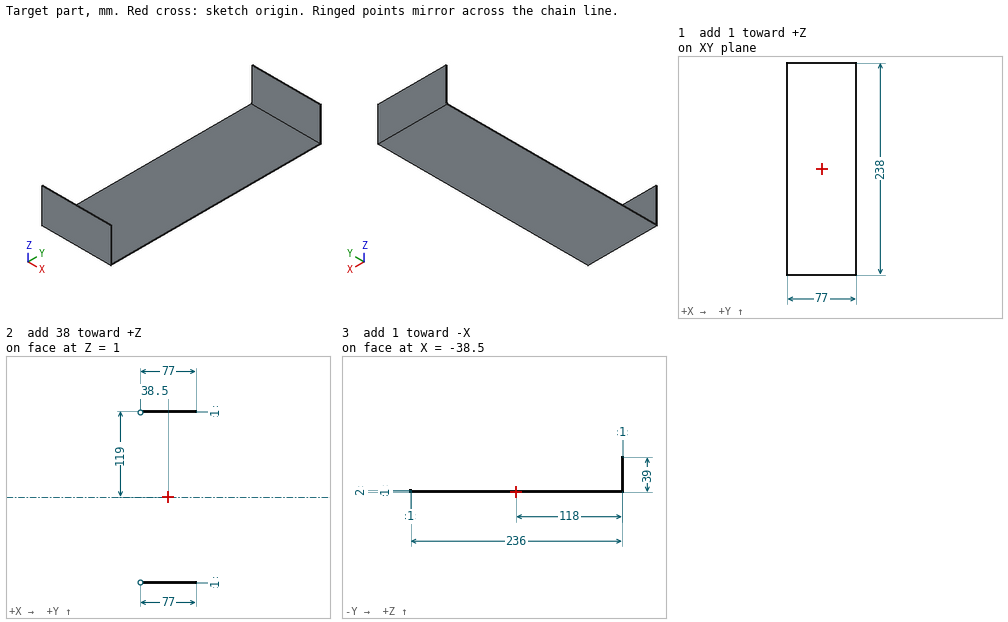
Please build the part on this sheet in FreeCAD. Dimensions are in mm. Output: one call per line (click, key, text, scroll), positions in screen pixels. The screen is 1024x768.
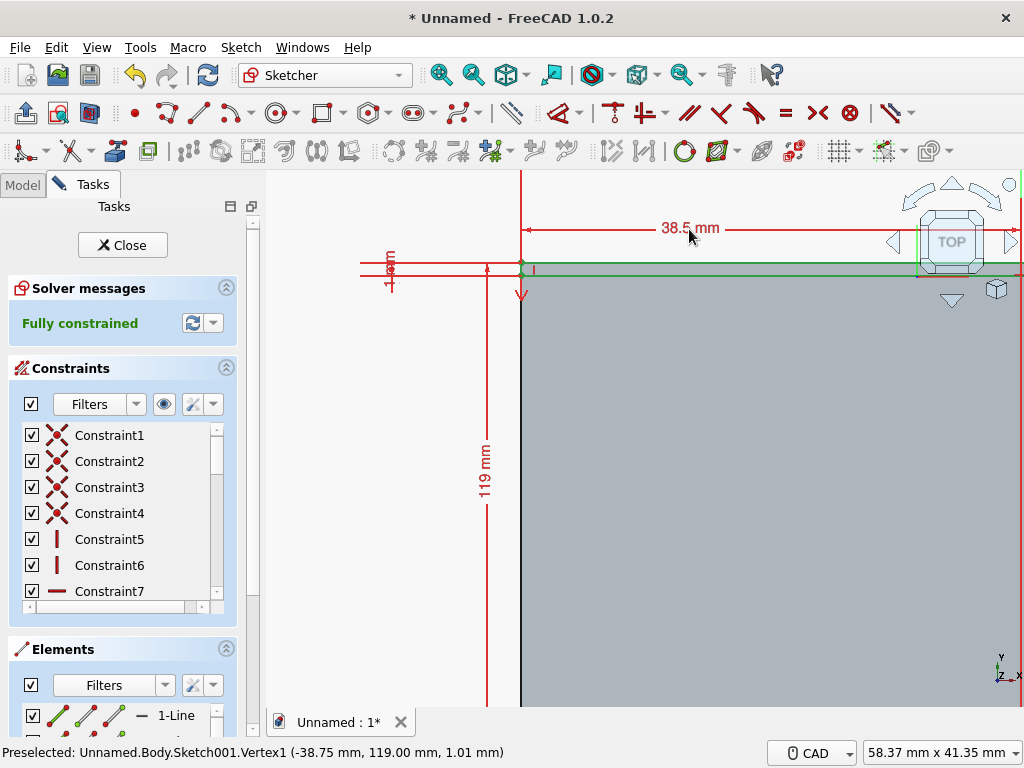
click(123, 245)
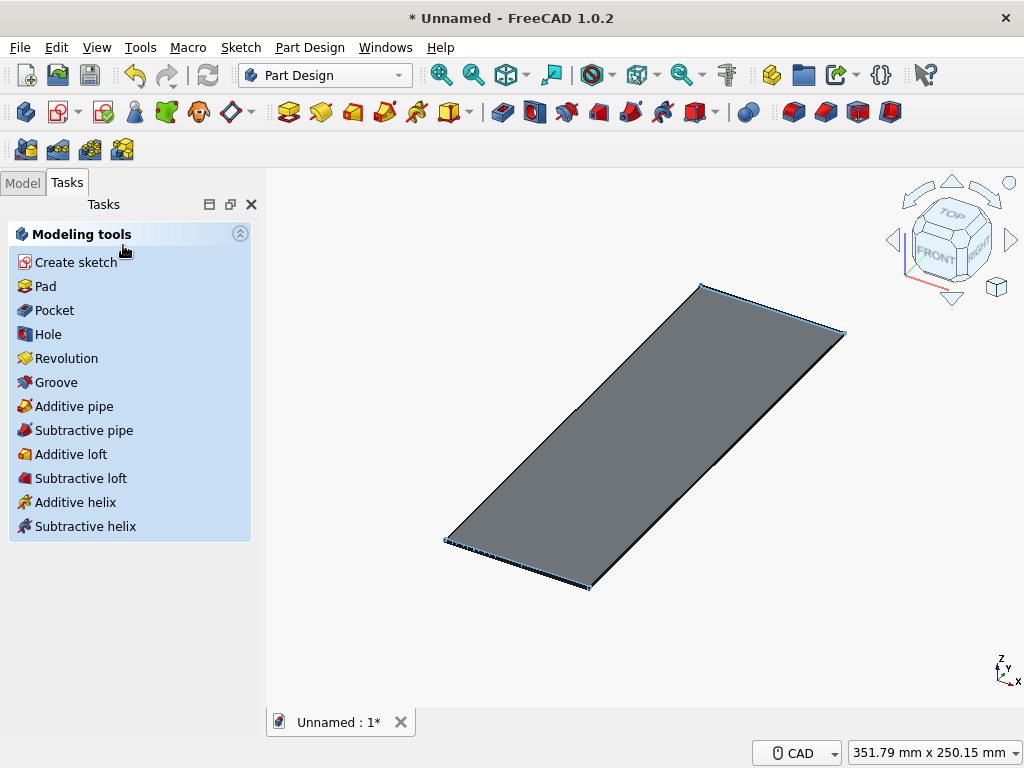
click(290, 112)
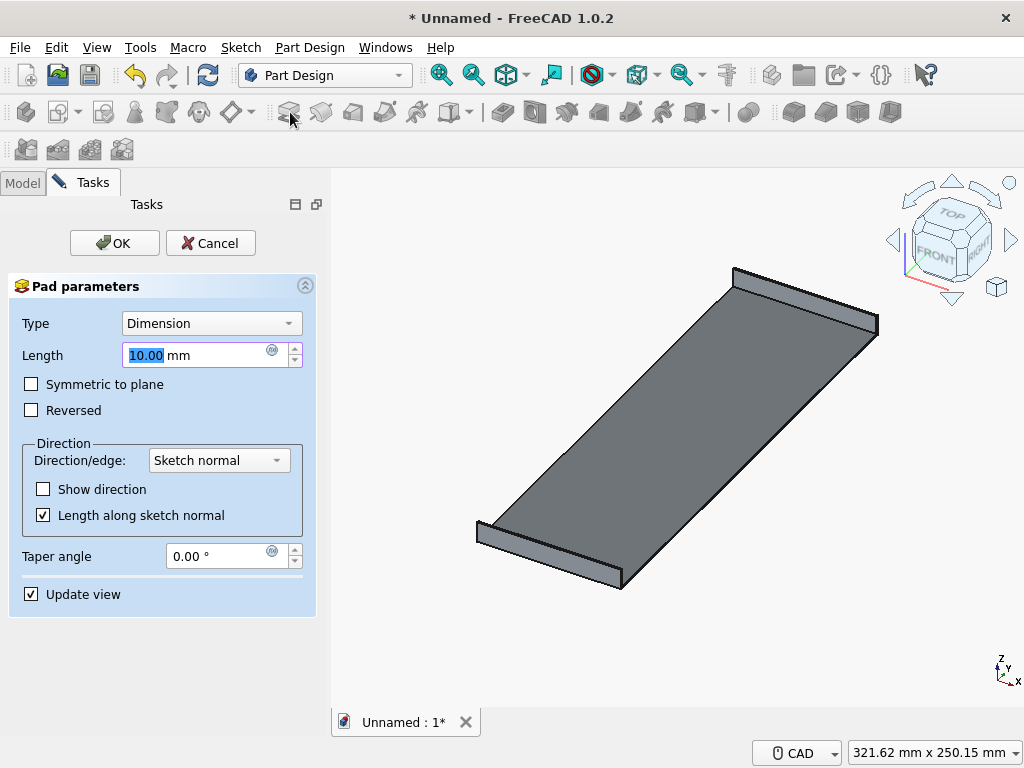
text(38)
key(Tab)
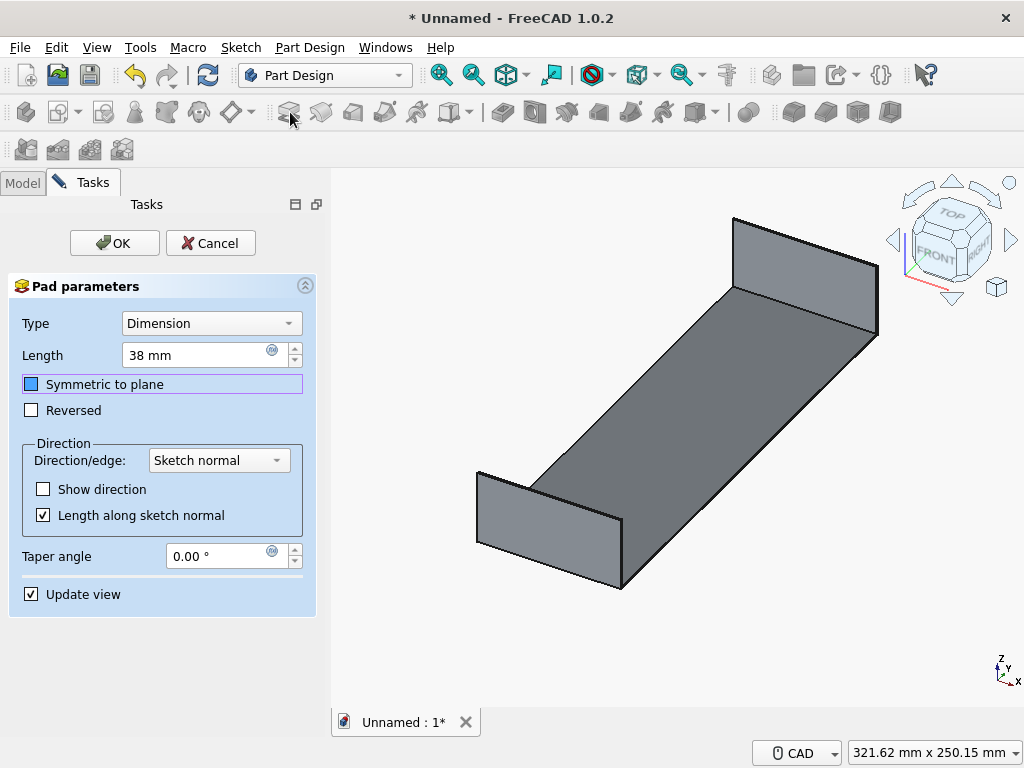
click(115, 243)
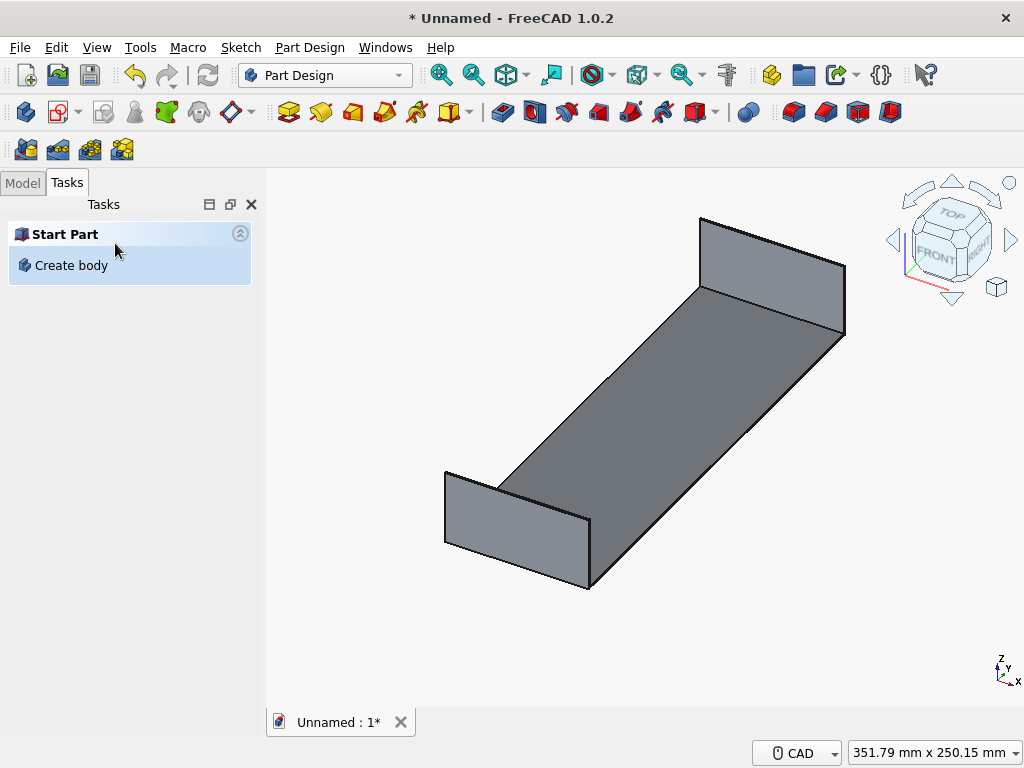
key(6)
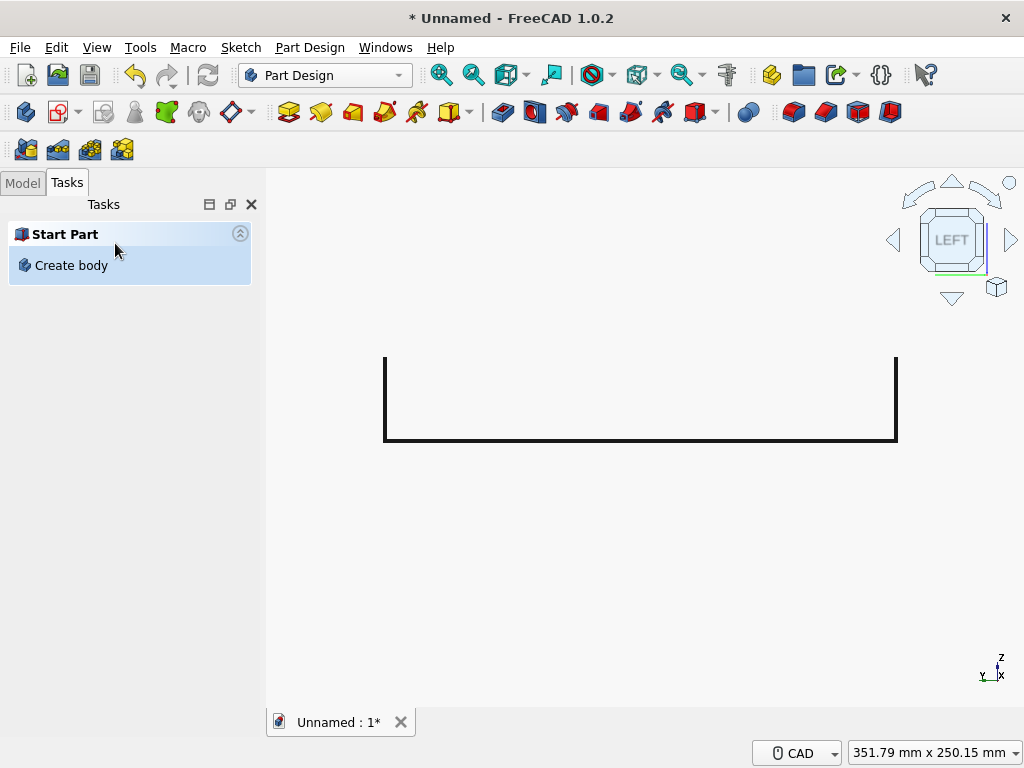
scroll(726, 439, up, 15)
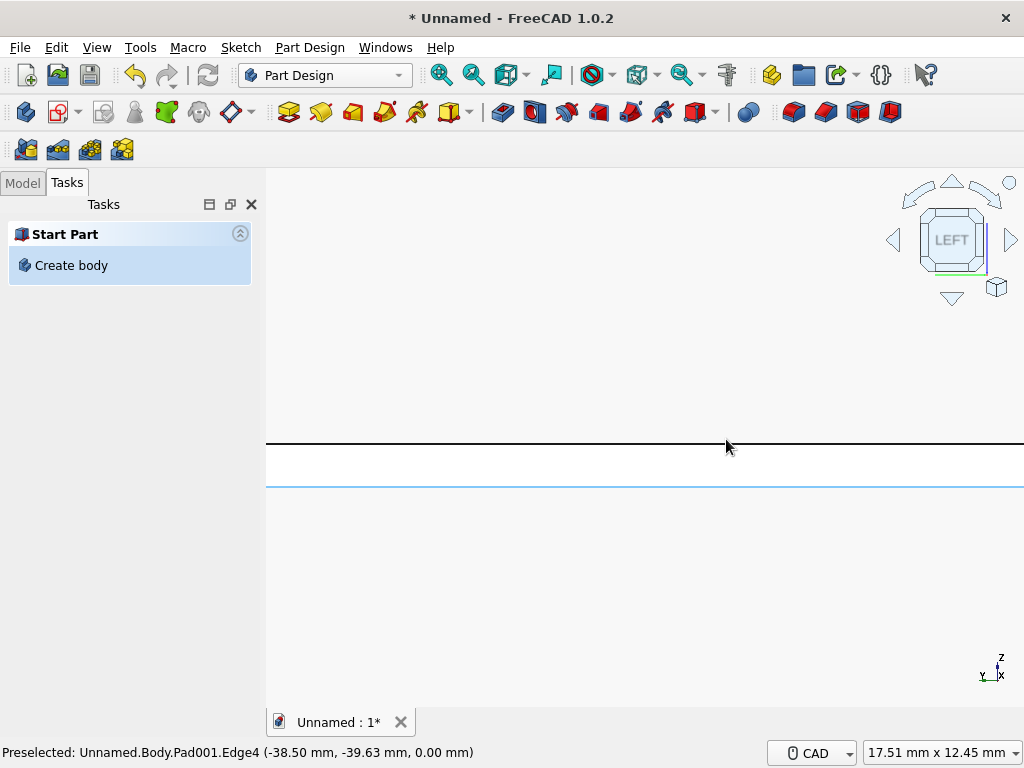
click(716, 457)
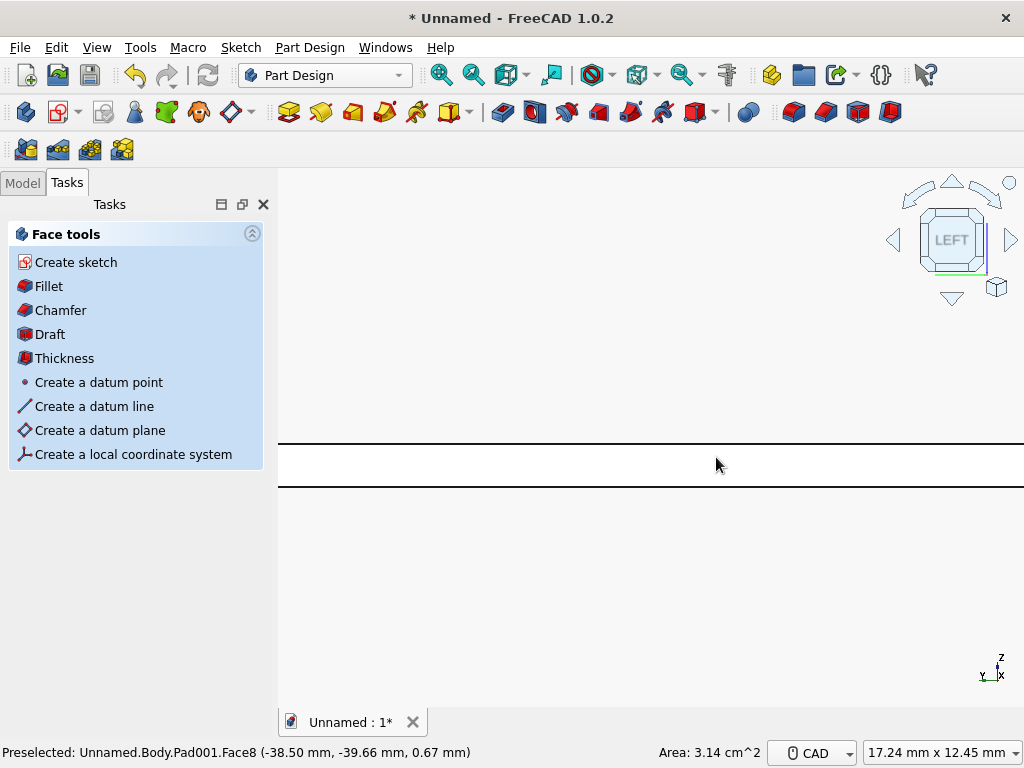
click(58, 112)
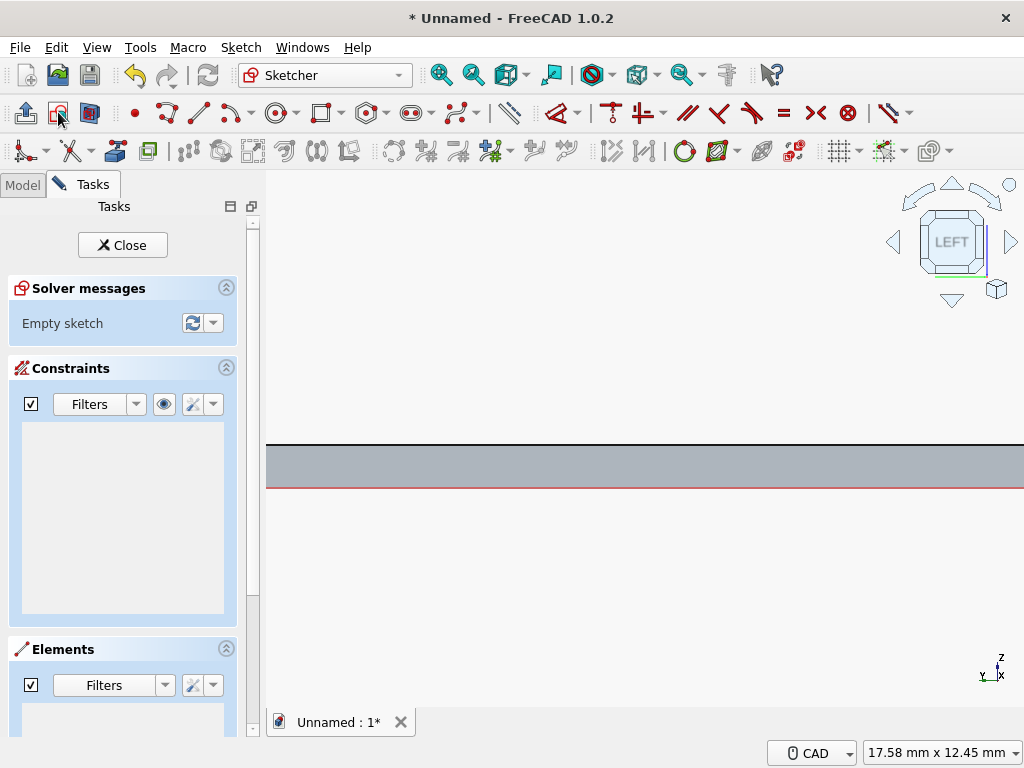
scroll(659, 480, down, 15)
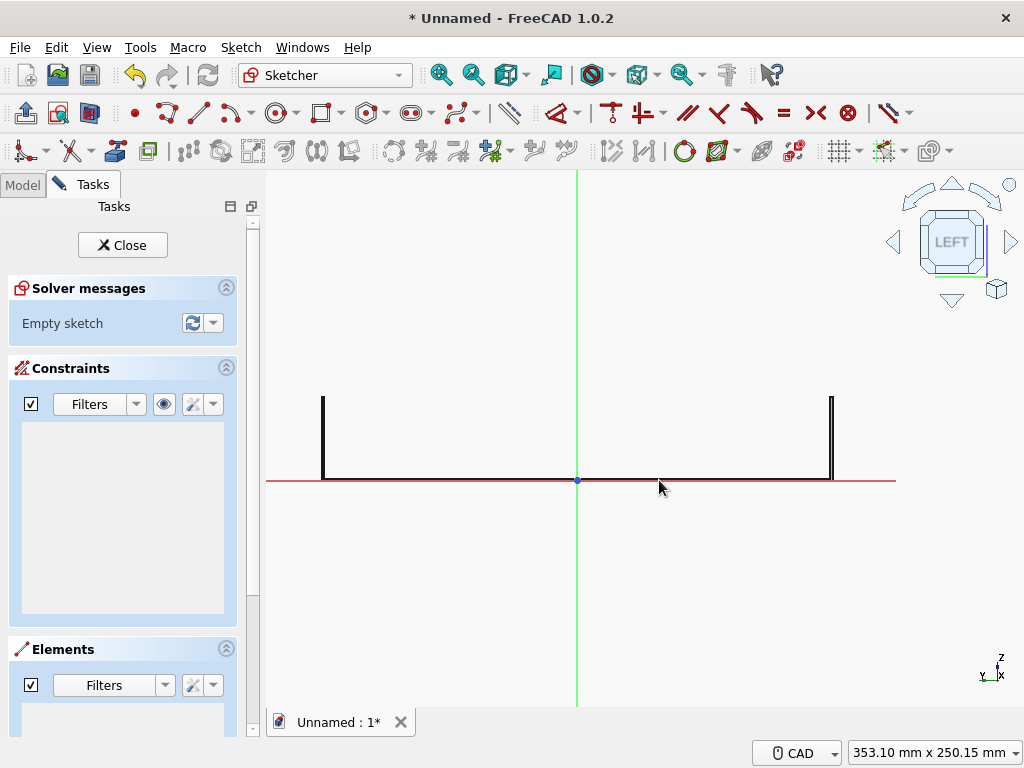
click(168, 114)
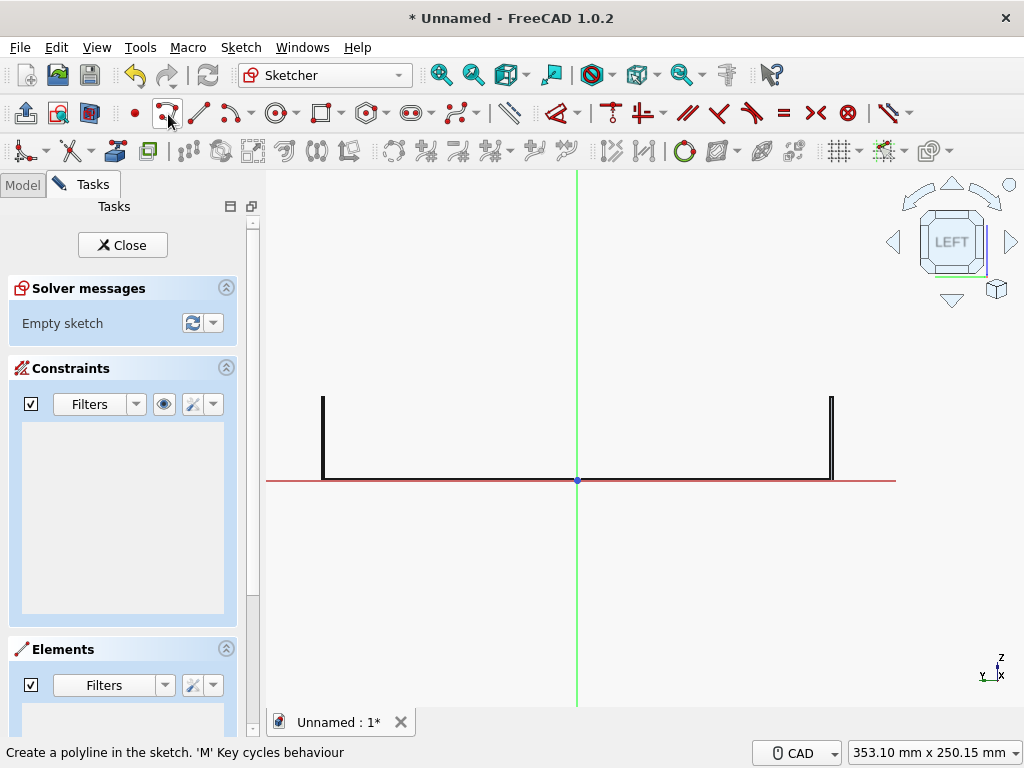
scroll(830, 479, up, 11)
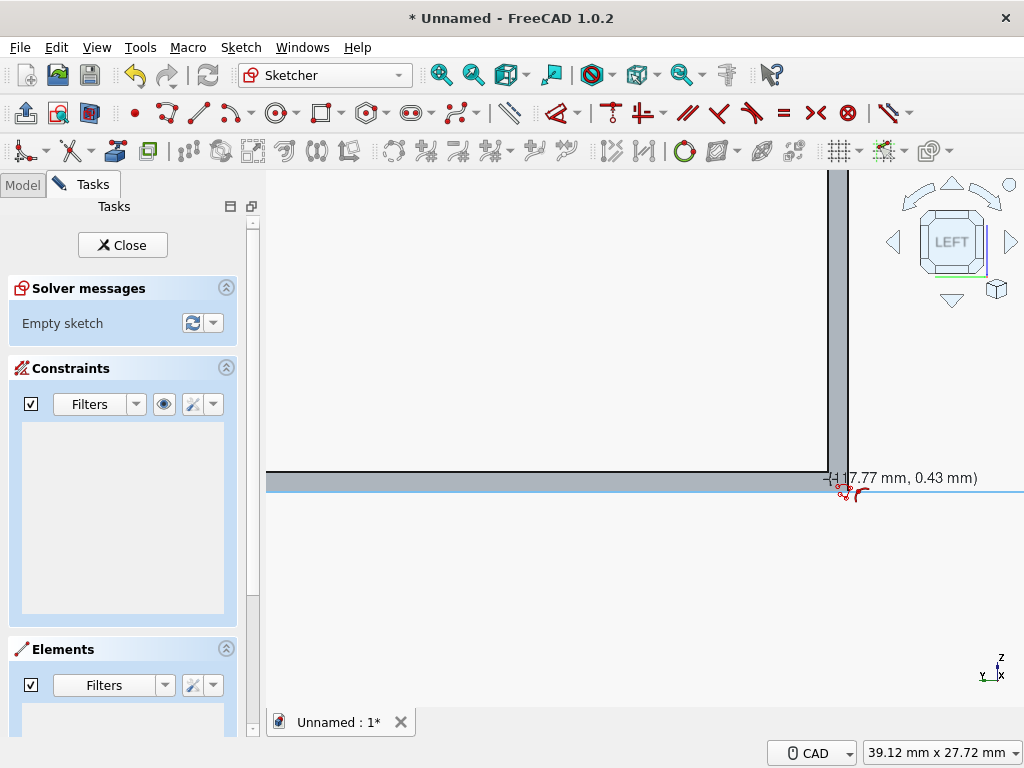
click(828, 472)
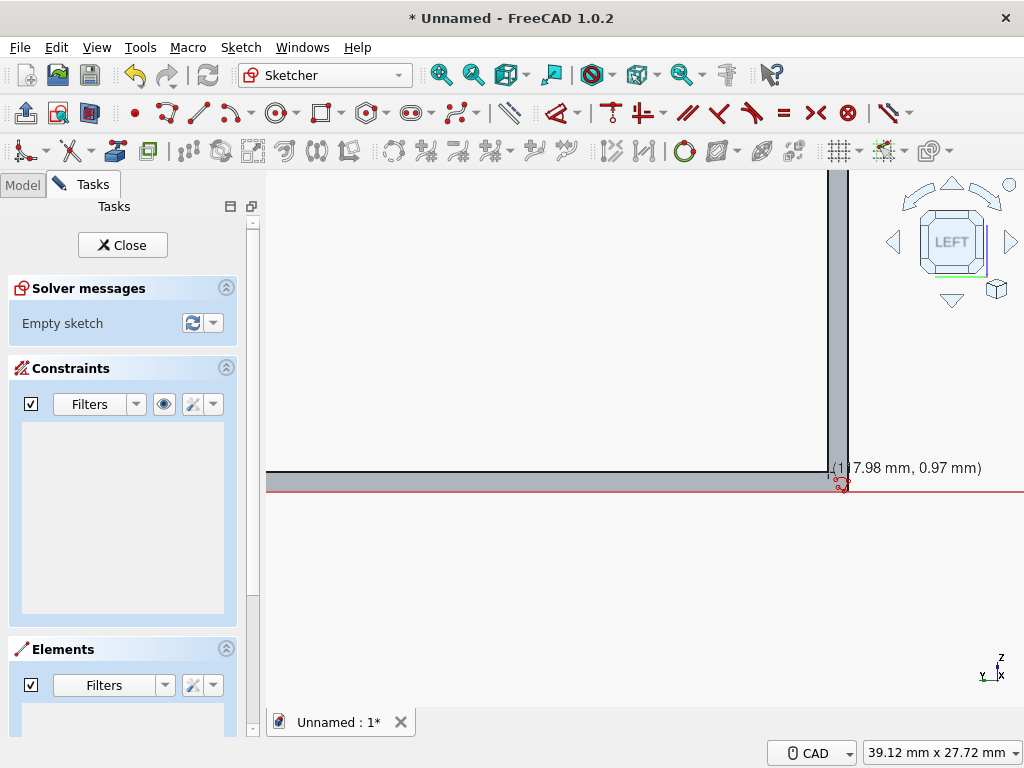
scroll(779, 471, down, 12)